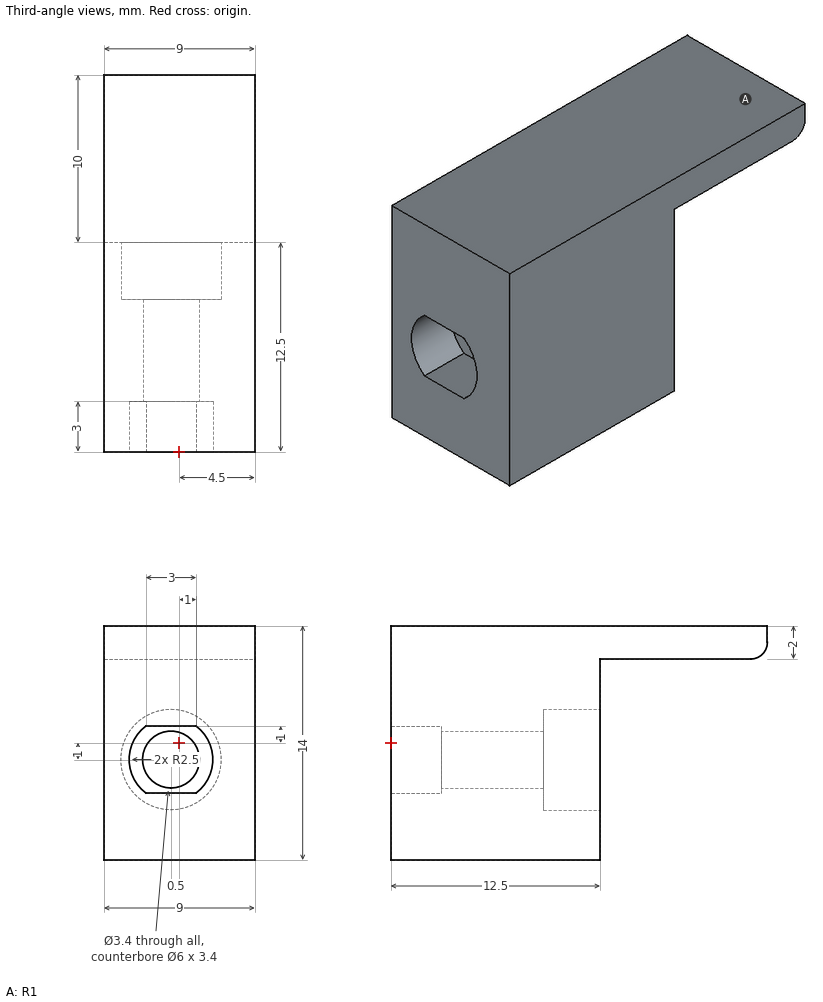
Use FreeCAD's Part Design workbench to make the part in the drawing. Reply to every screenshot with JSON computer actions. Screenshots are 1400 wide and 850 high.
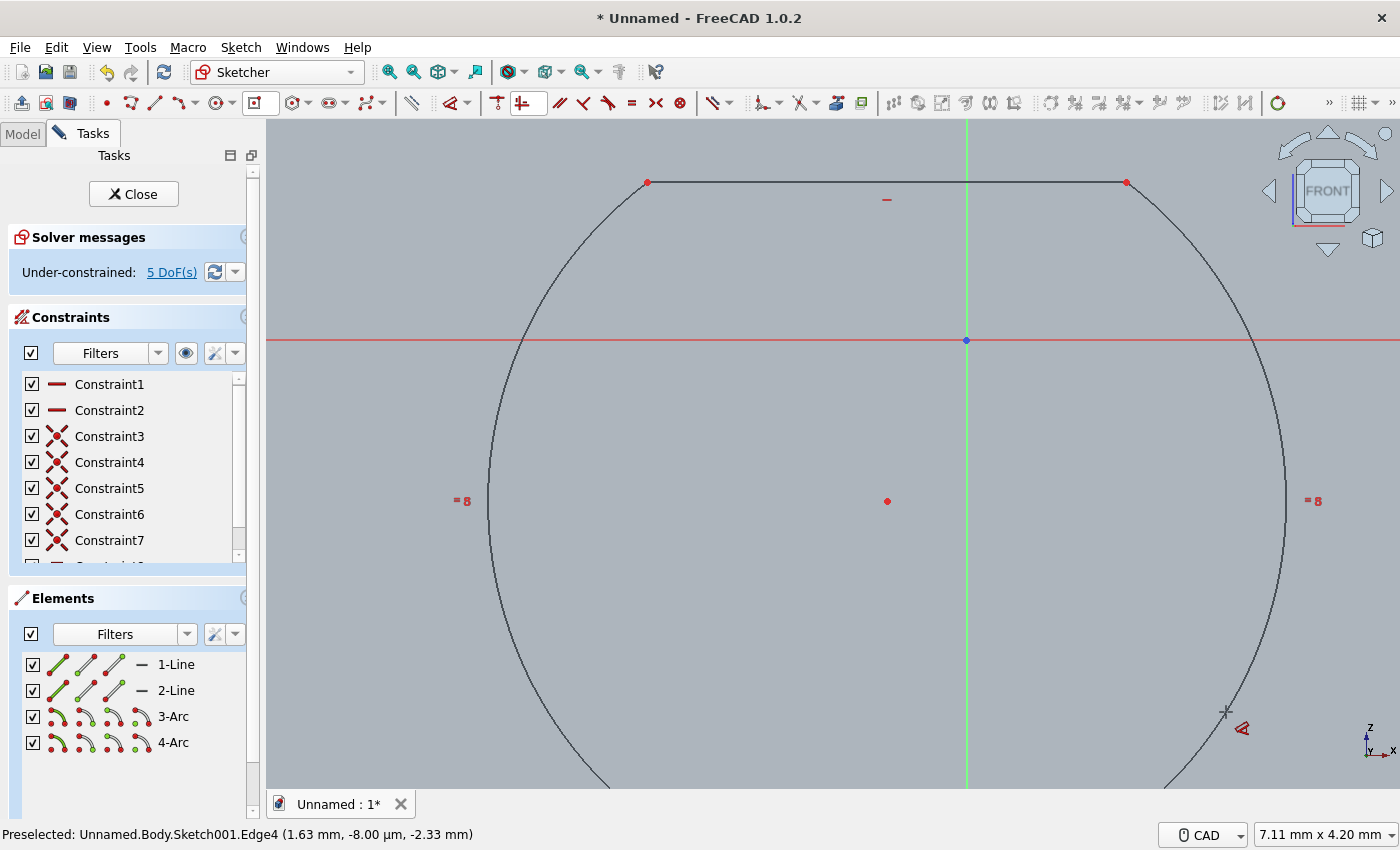
{"action": "left_click", "coordinate": [515, 357]}
{"action": "left_click", "coordinate": [609, 172]}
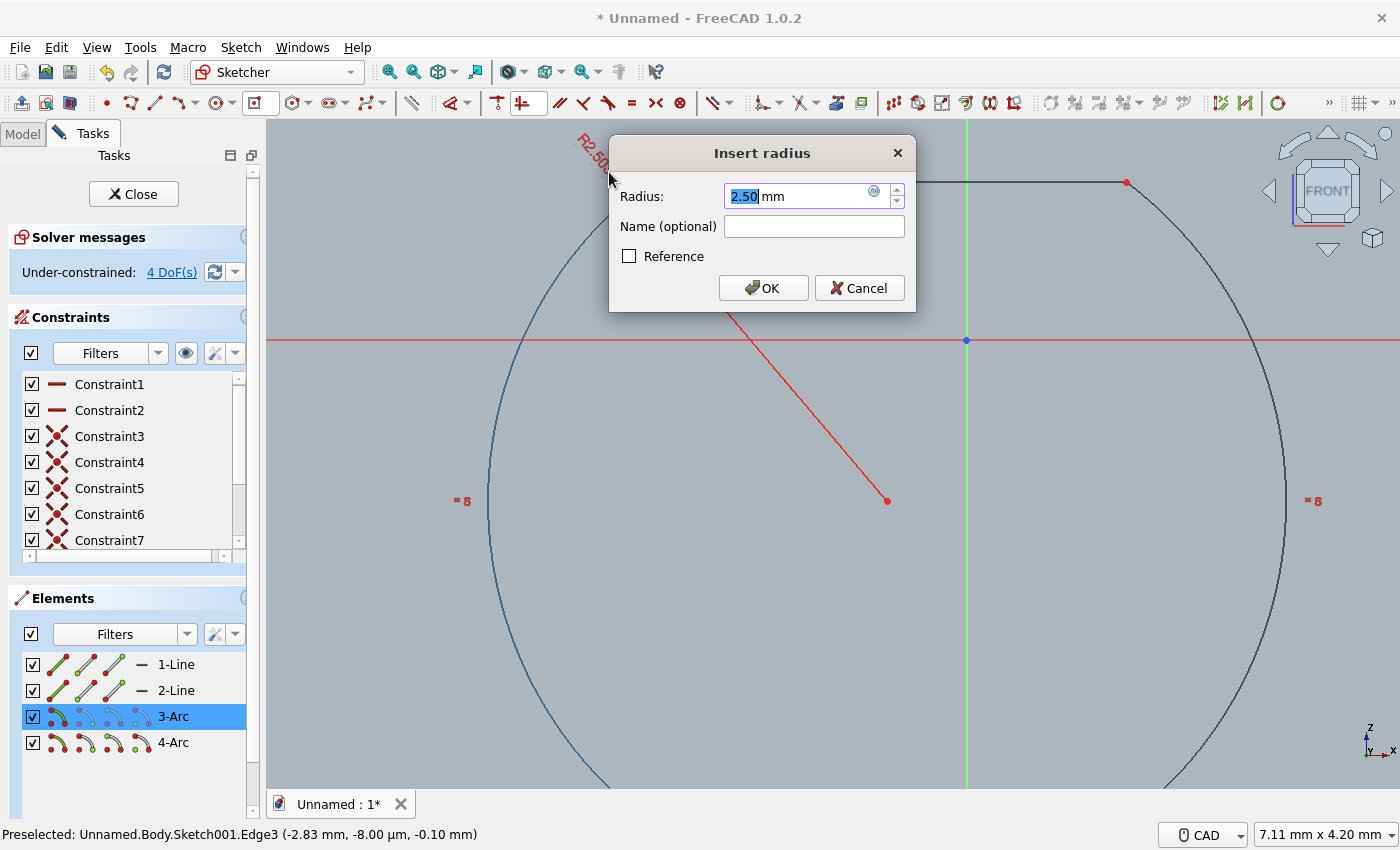
{"action": "type", "text": "2.5"}
{"action": "key", "text": "Return"}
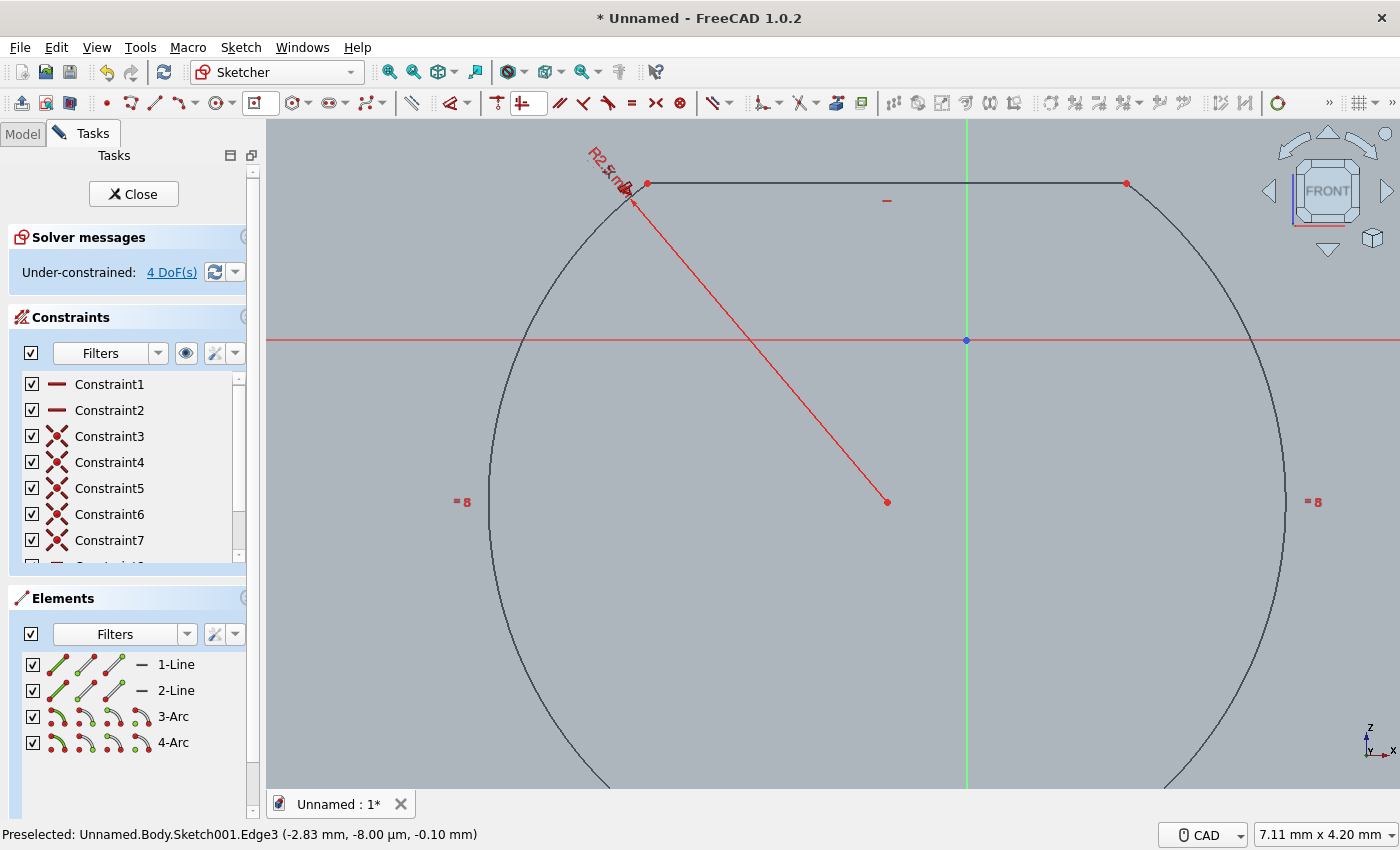
{"action": "left_click", "coordinate": [983, 183]}
{"action": "left_click", "coordinate": [887, 149]}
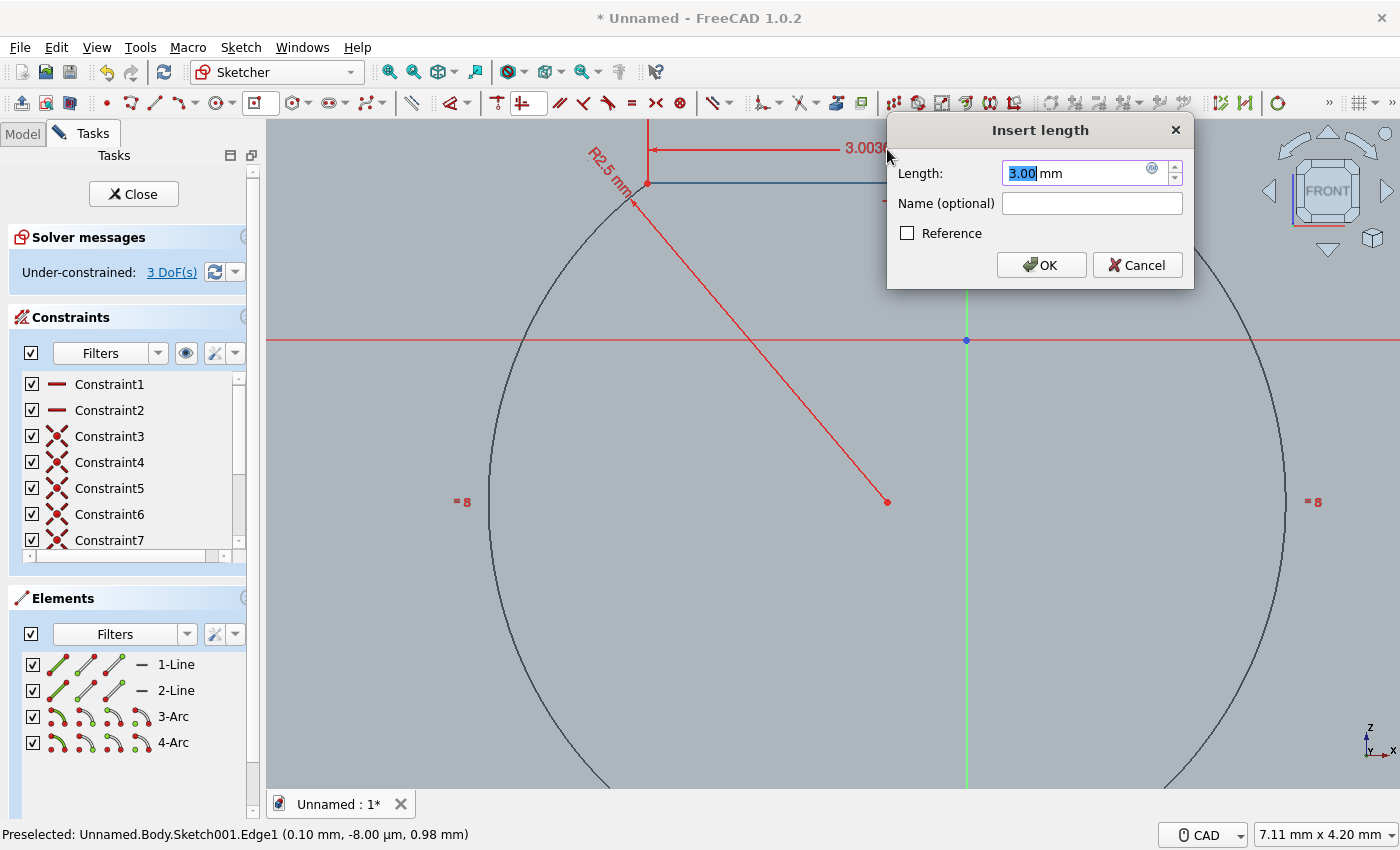
{"action": "type", "text": "3"}
{"action": "key", "text": "Return"}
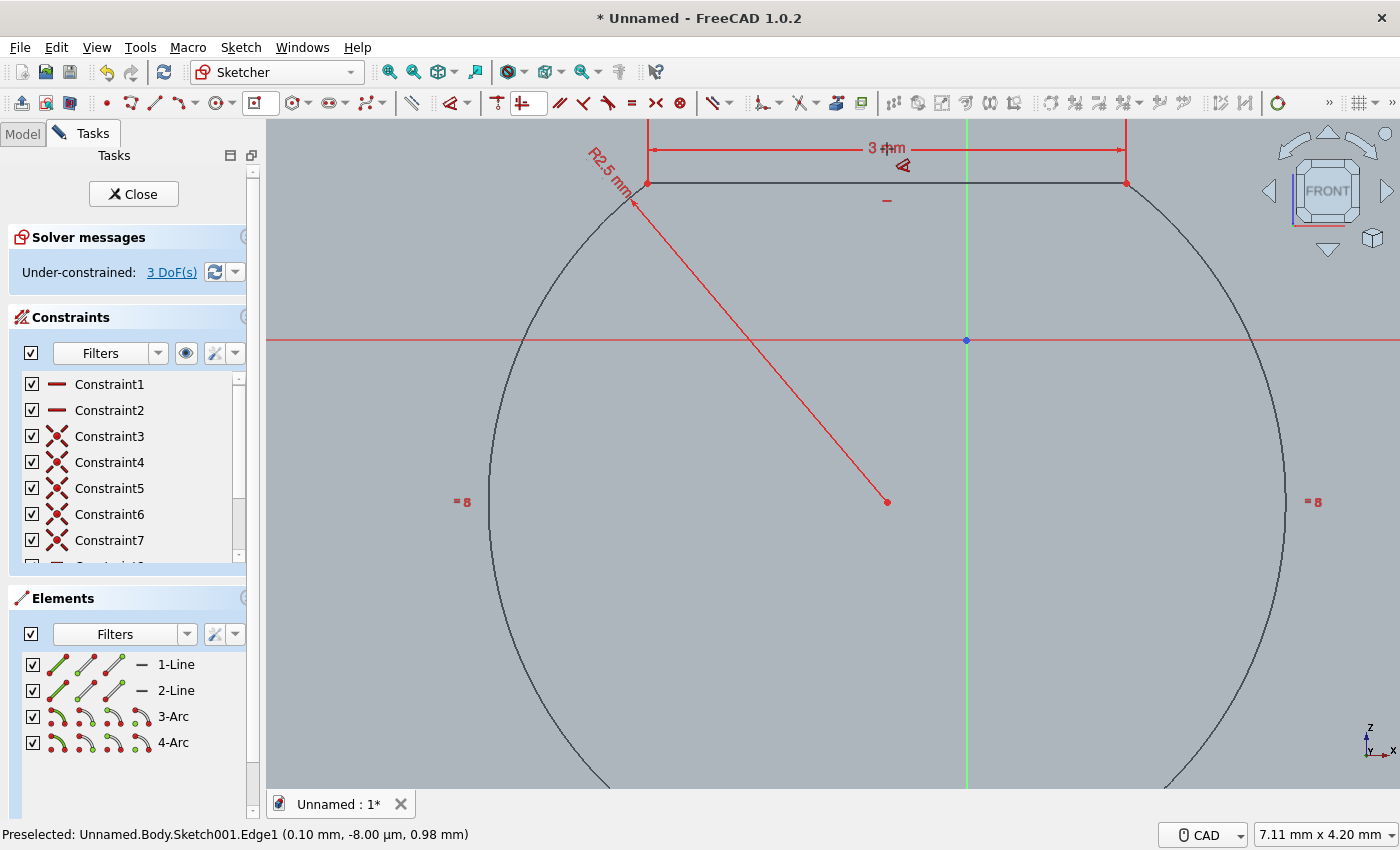
{"action": "scroll", "coordinate": [515, 361], "scroll_direction": "down", "scroll_amount": 2}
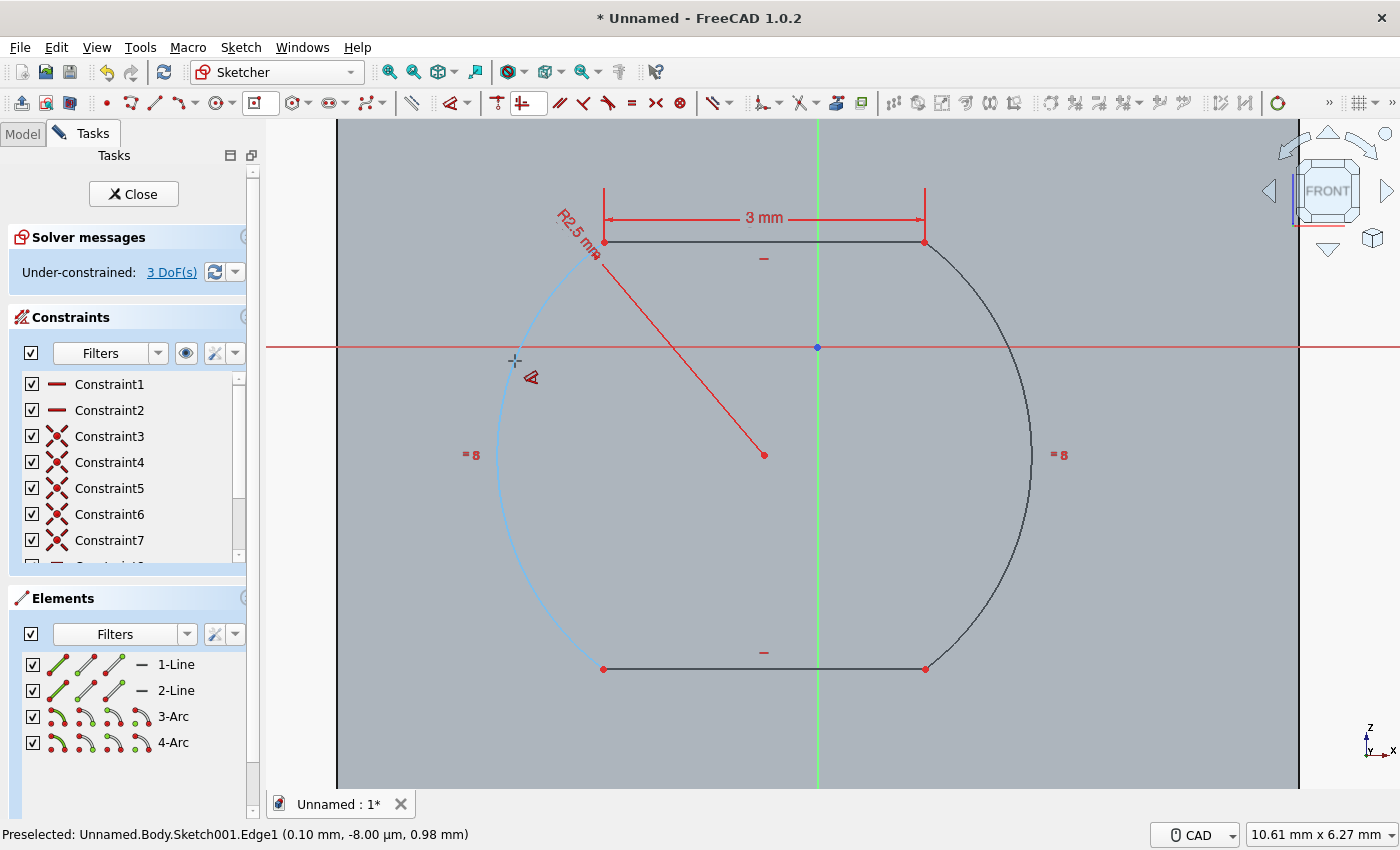
{"action": "left_click", "coordinate": [700, 669]}
{"action": "left_click", "coordinate": [764, 703]}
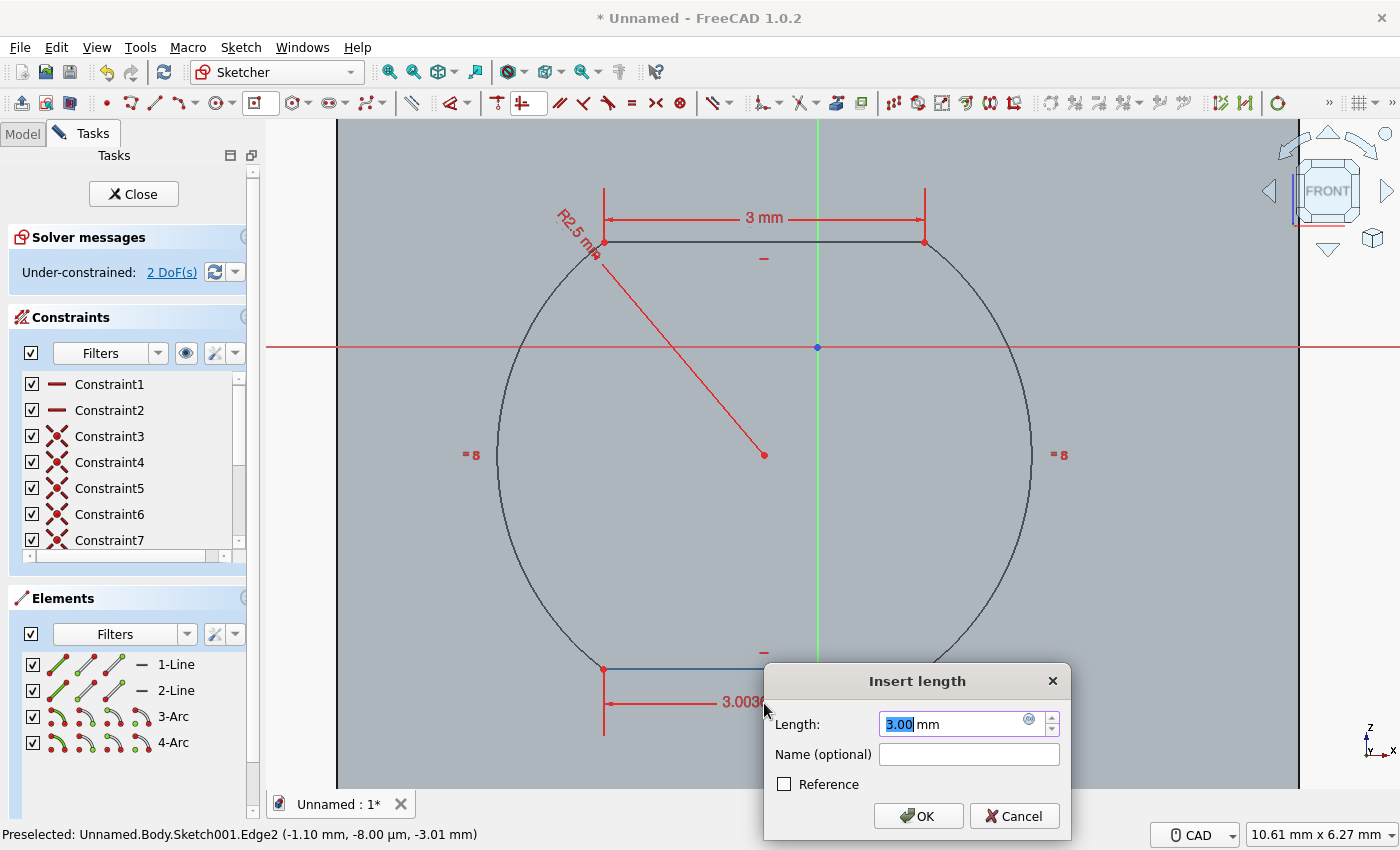
{"action": "type", "text": "3"}
{"action": "key", "text": "Return"}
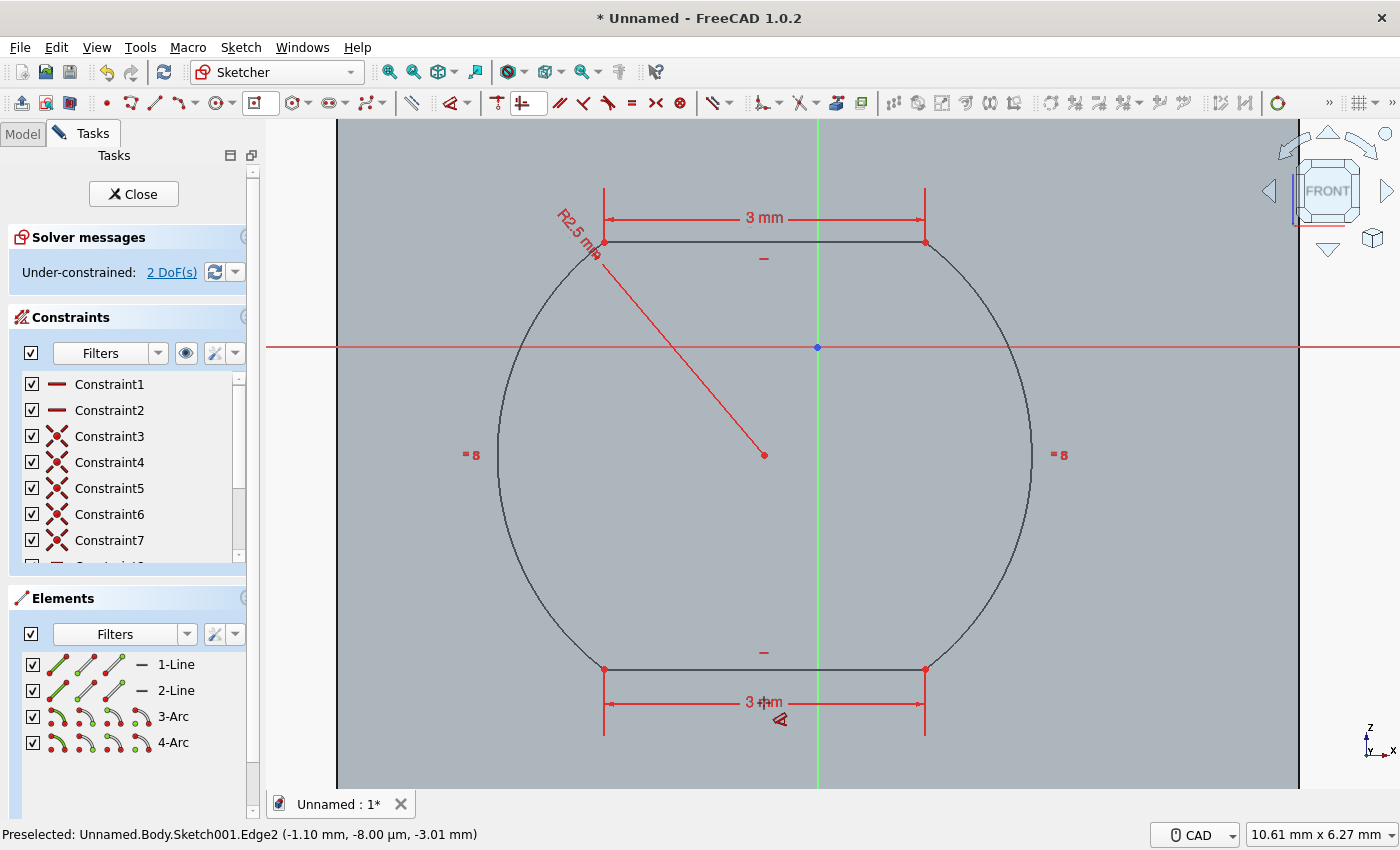
{"action": "left_click", "coordinate": [925, 242]}
{"action": "left_click", "coordinate": [871, 208]}